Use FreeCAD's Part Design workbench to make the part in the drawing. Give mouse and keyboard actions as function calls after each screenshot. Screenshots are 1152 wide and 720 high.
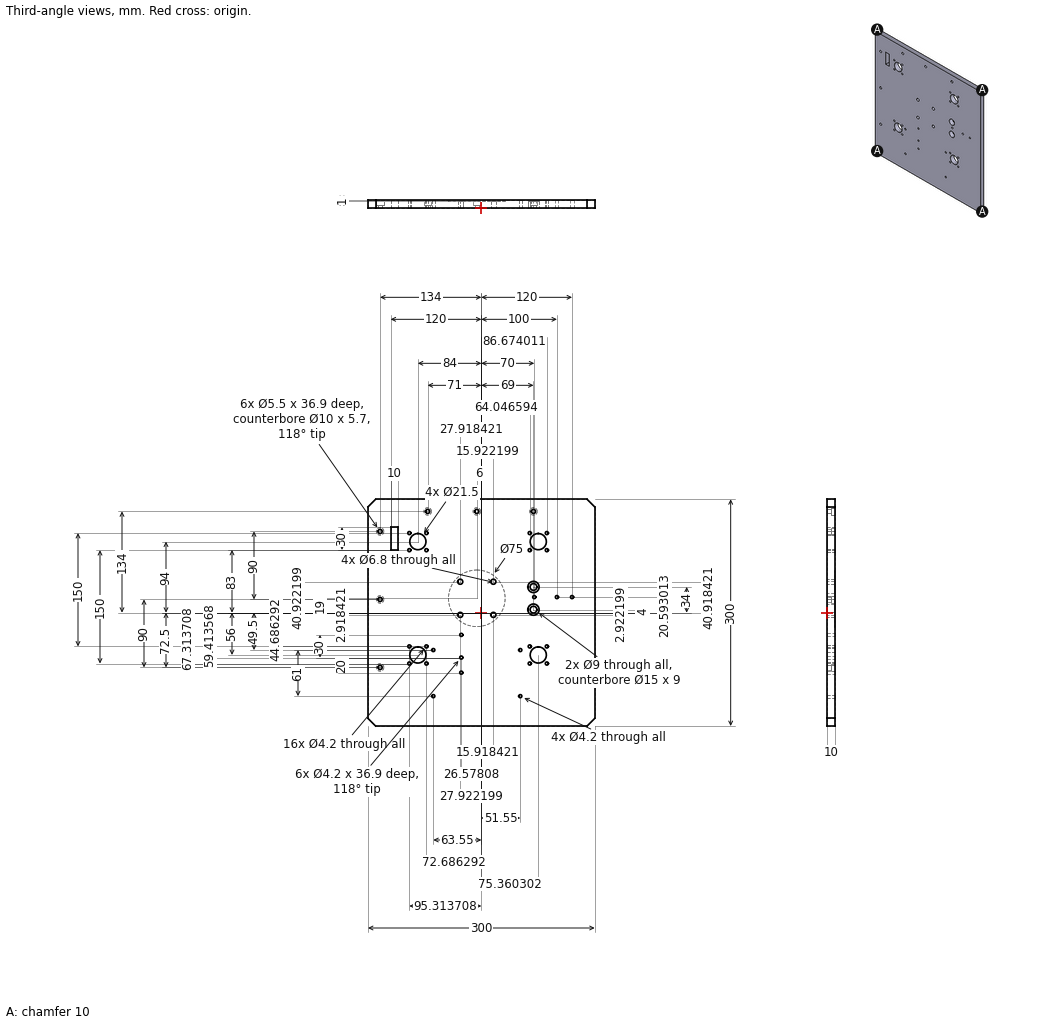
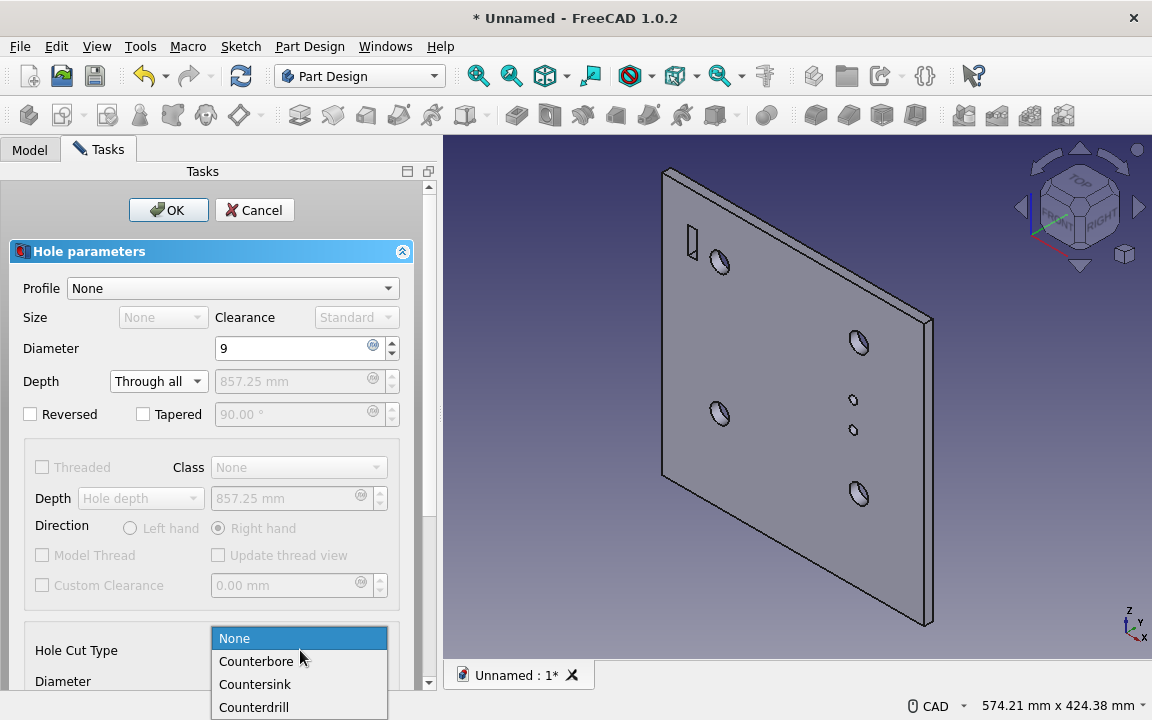
click(298, 662)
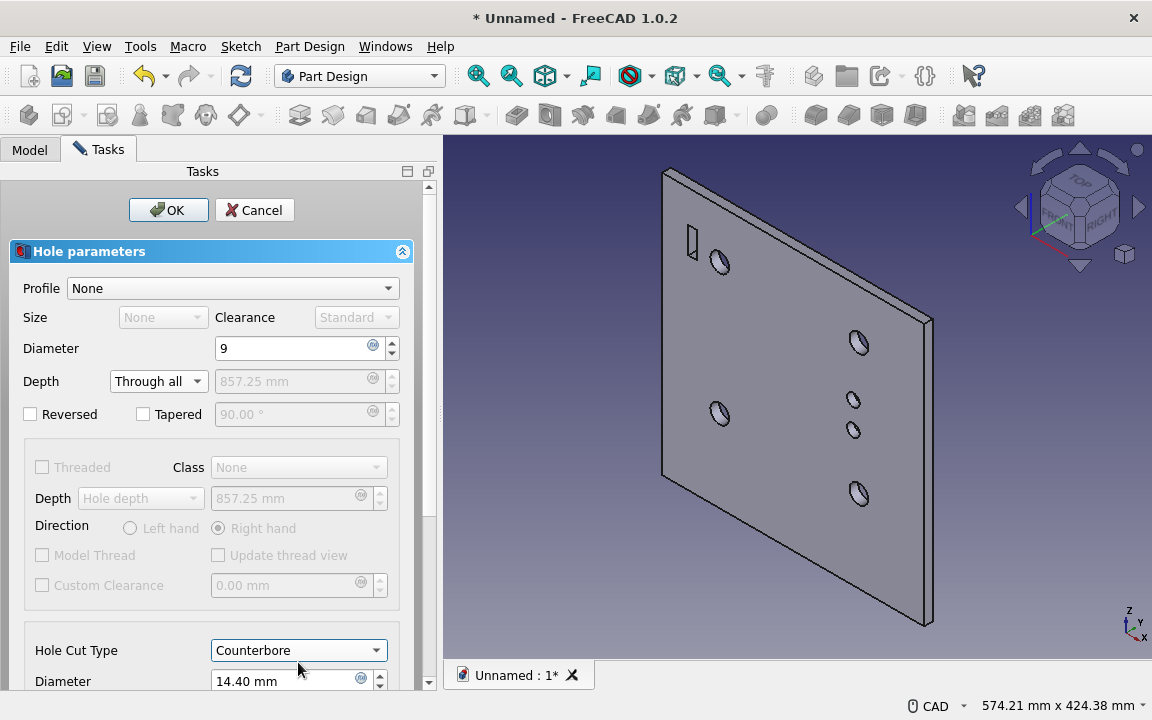
scroll(429, 436, down, 2)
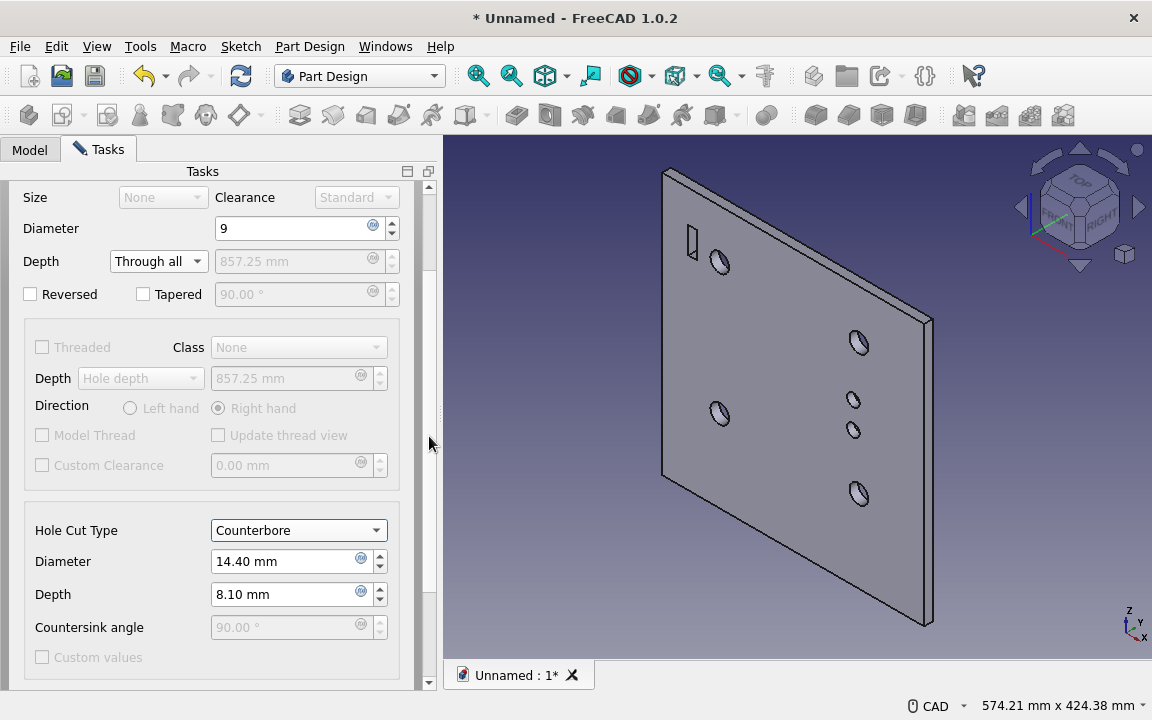
triple_click(292, 562)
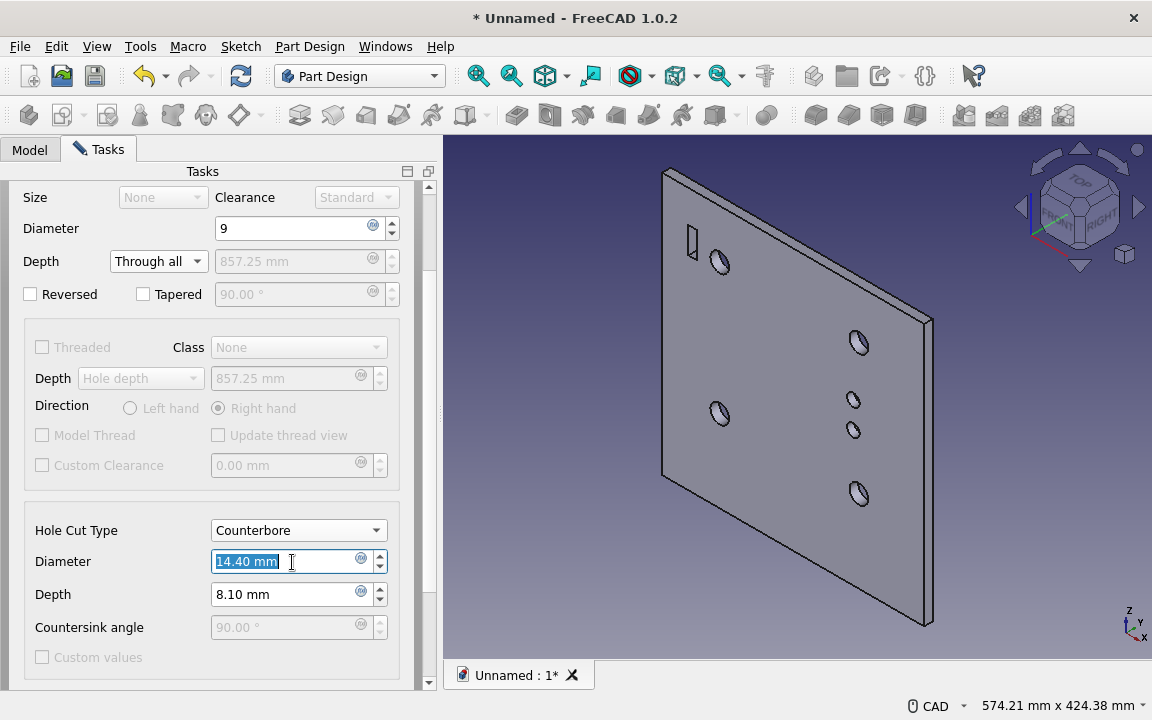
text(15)
key(Tab)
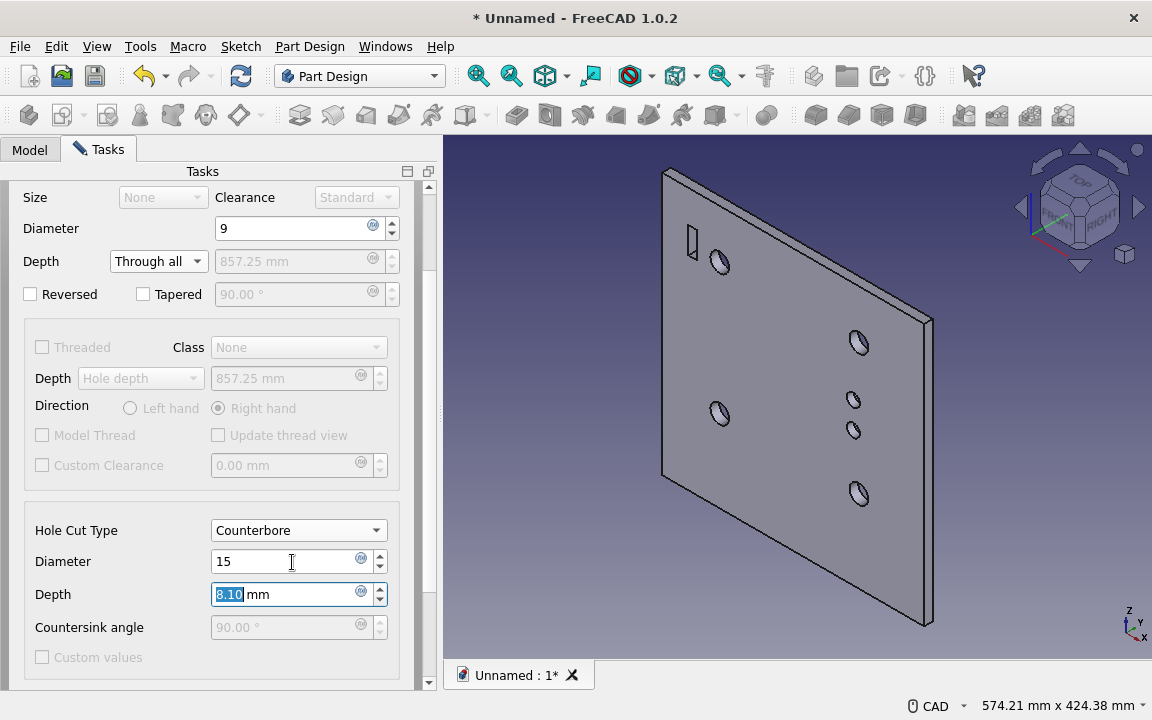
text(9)
key(Tab)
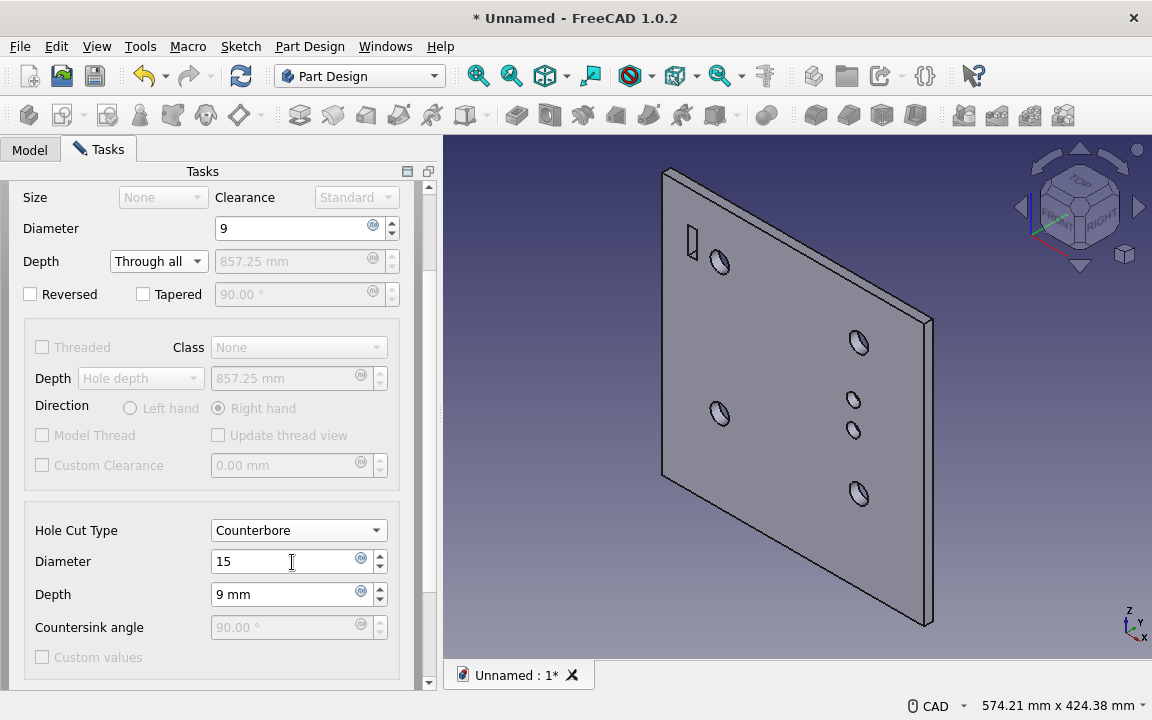
scroll(429, 436, up, 3)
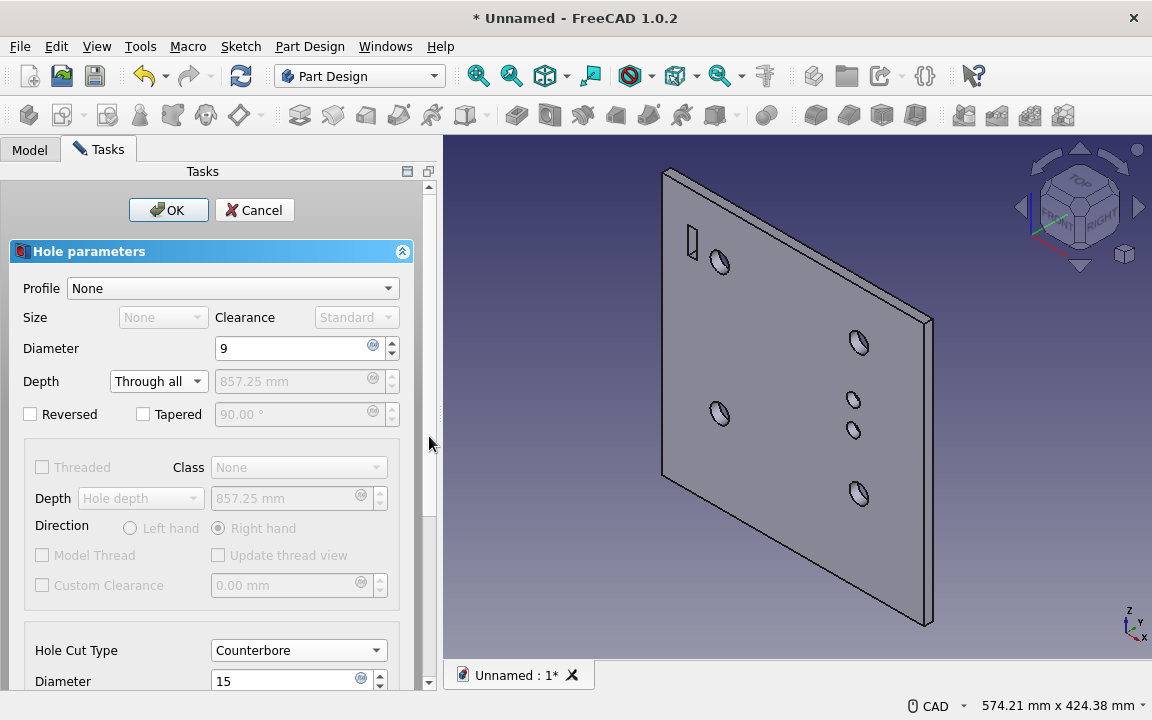
click(169, 210)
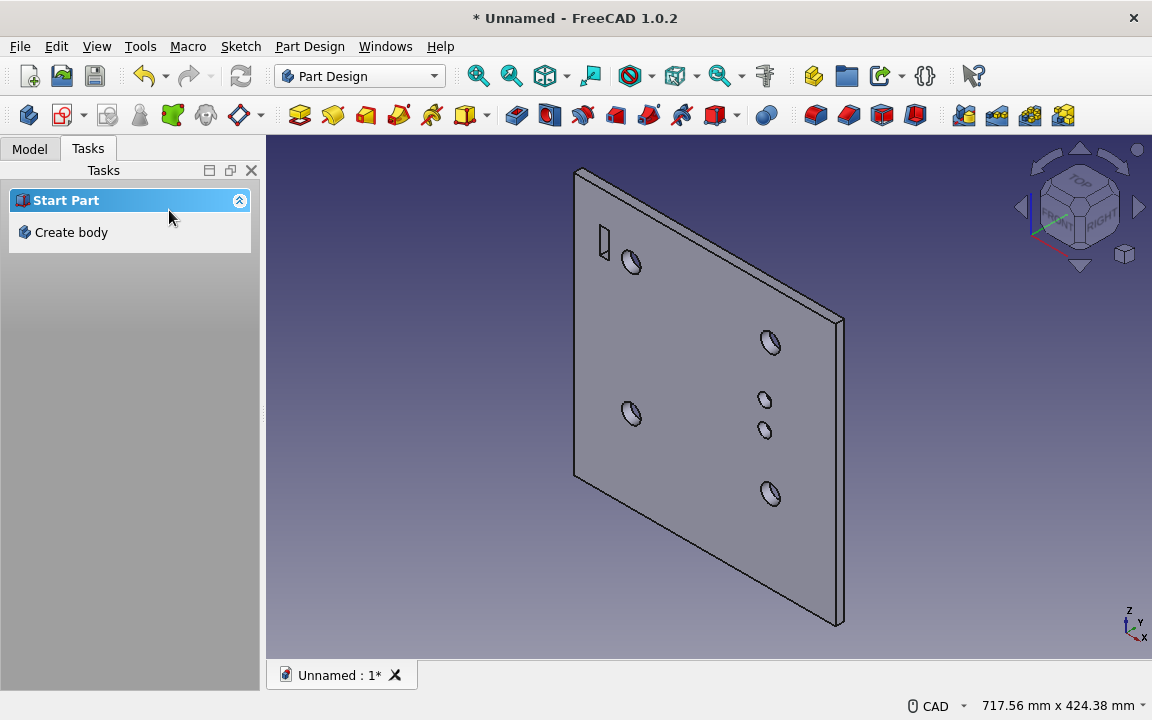
key(4)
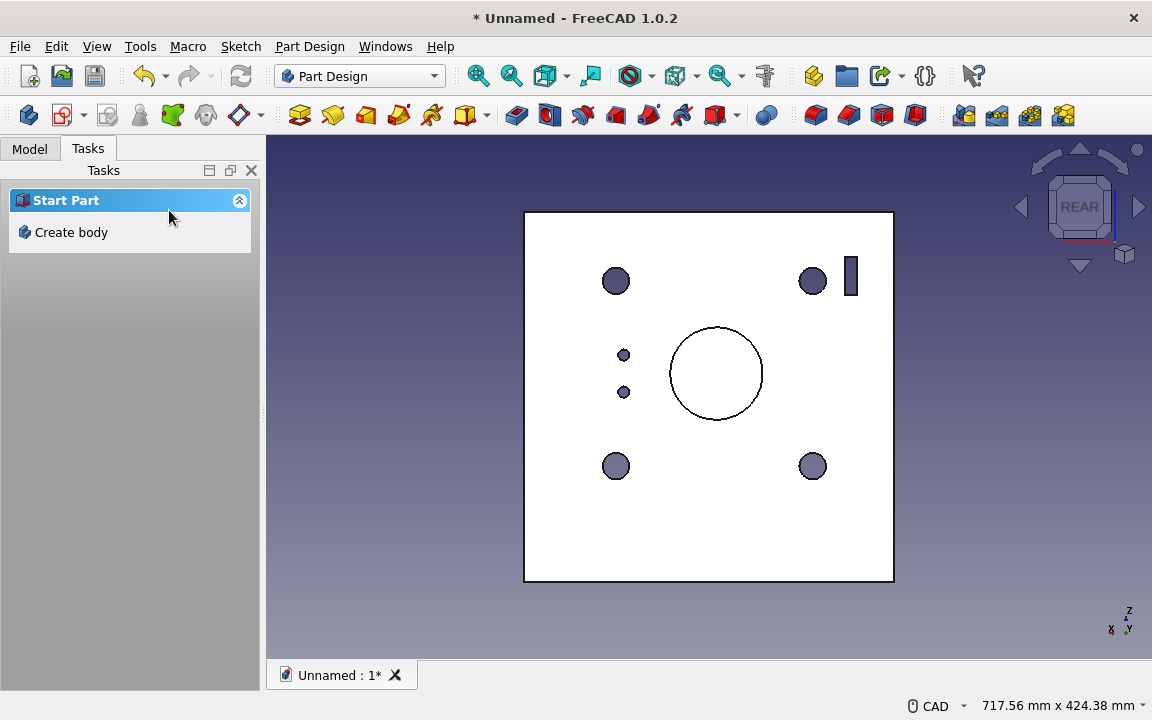
click(709, 502)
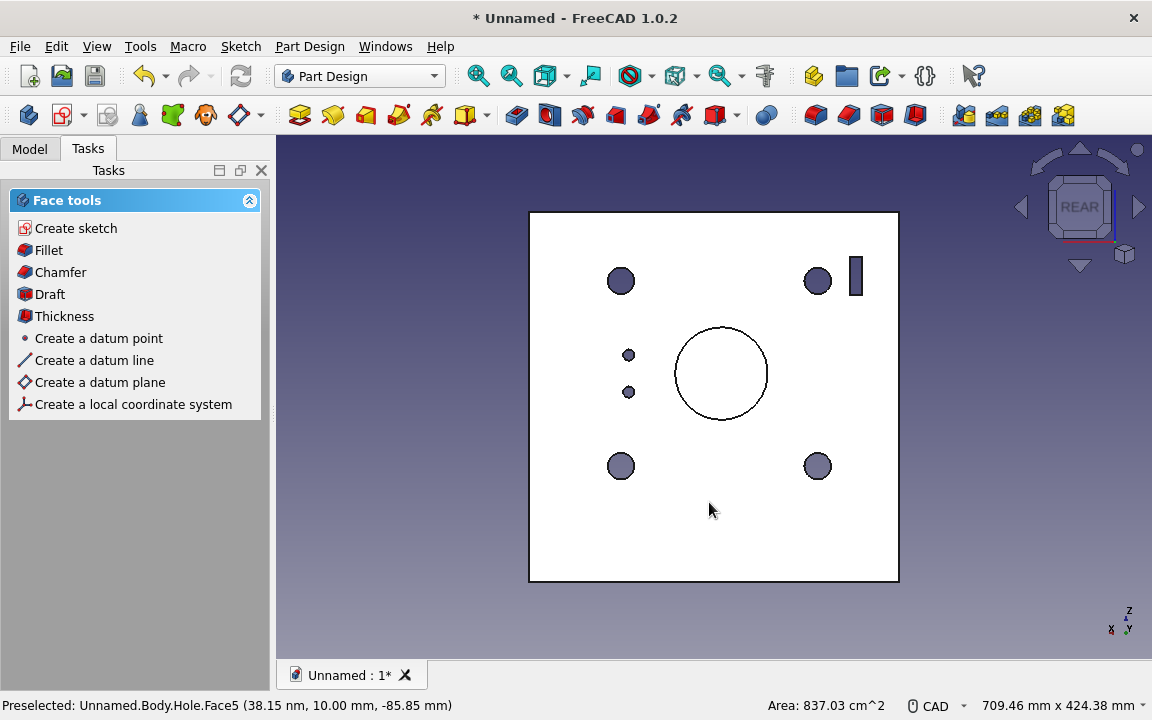
click(62, 116)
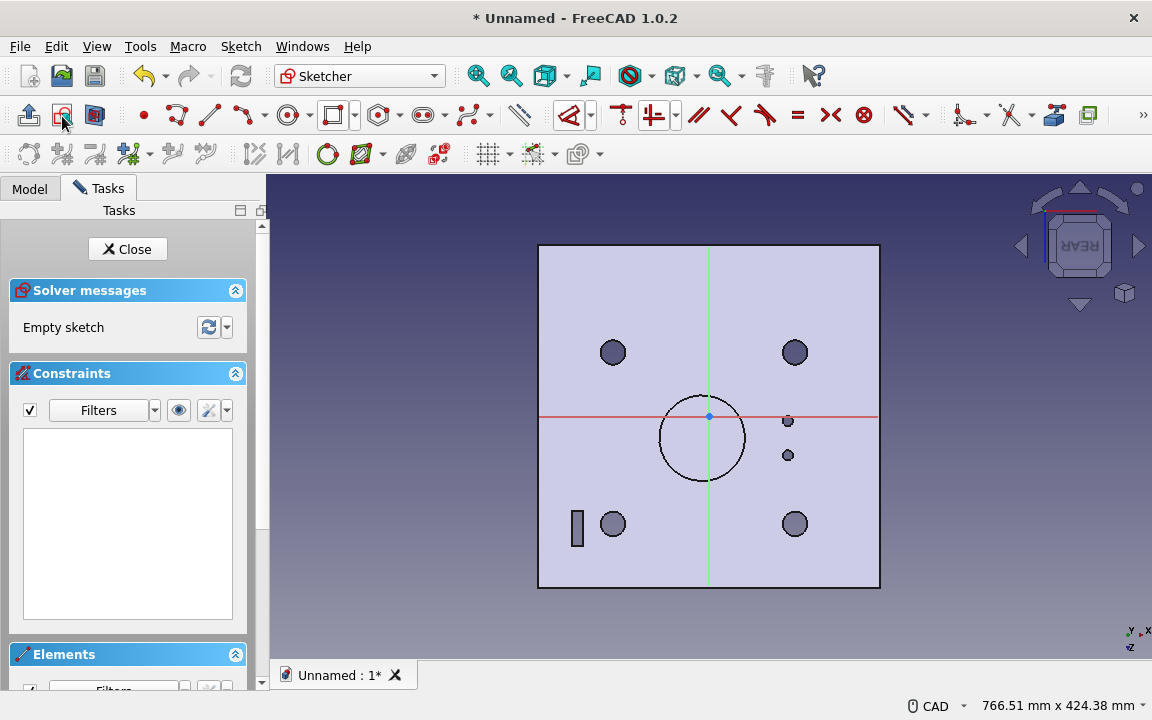
scroll(718, 444, up, 8)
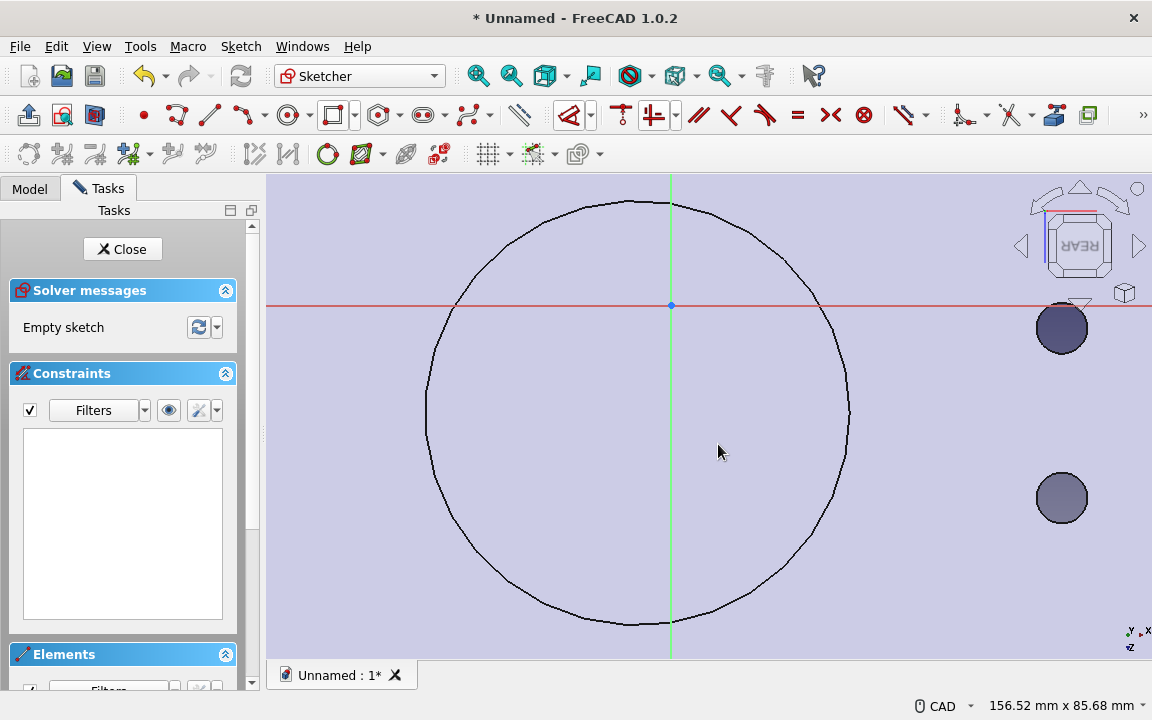
click(288, 116)